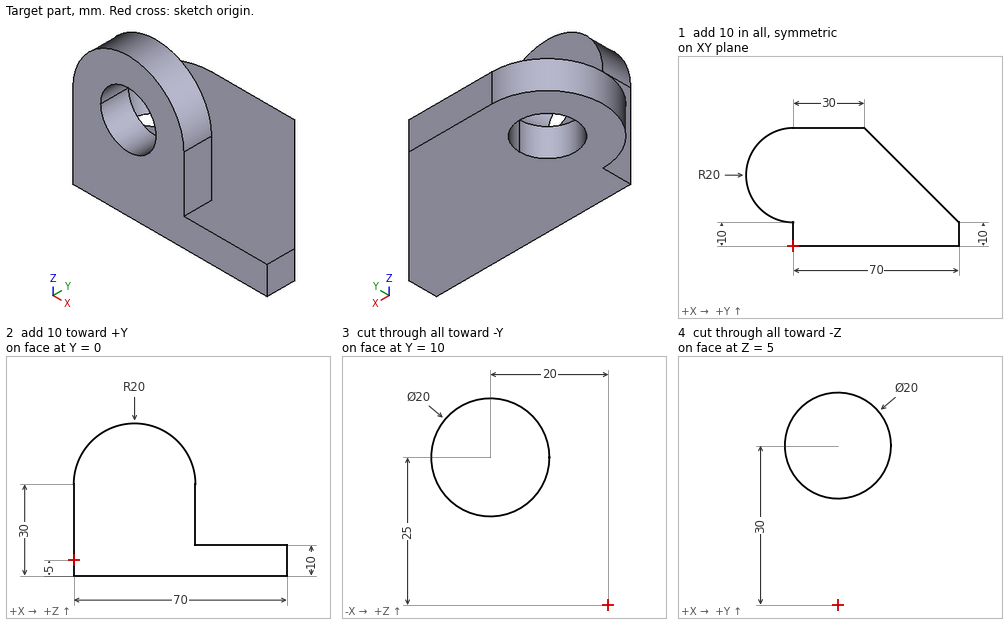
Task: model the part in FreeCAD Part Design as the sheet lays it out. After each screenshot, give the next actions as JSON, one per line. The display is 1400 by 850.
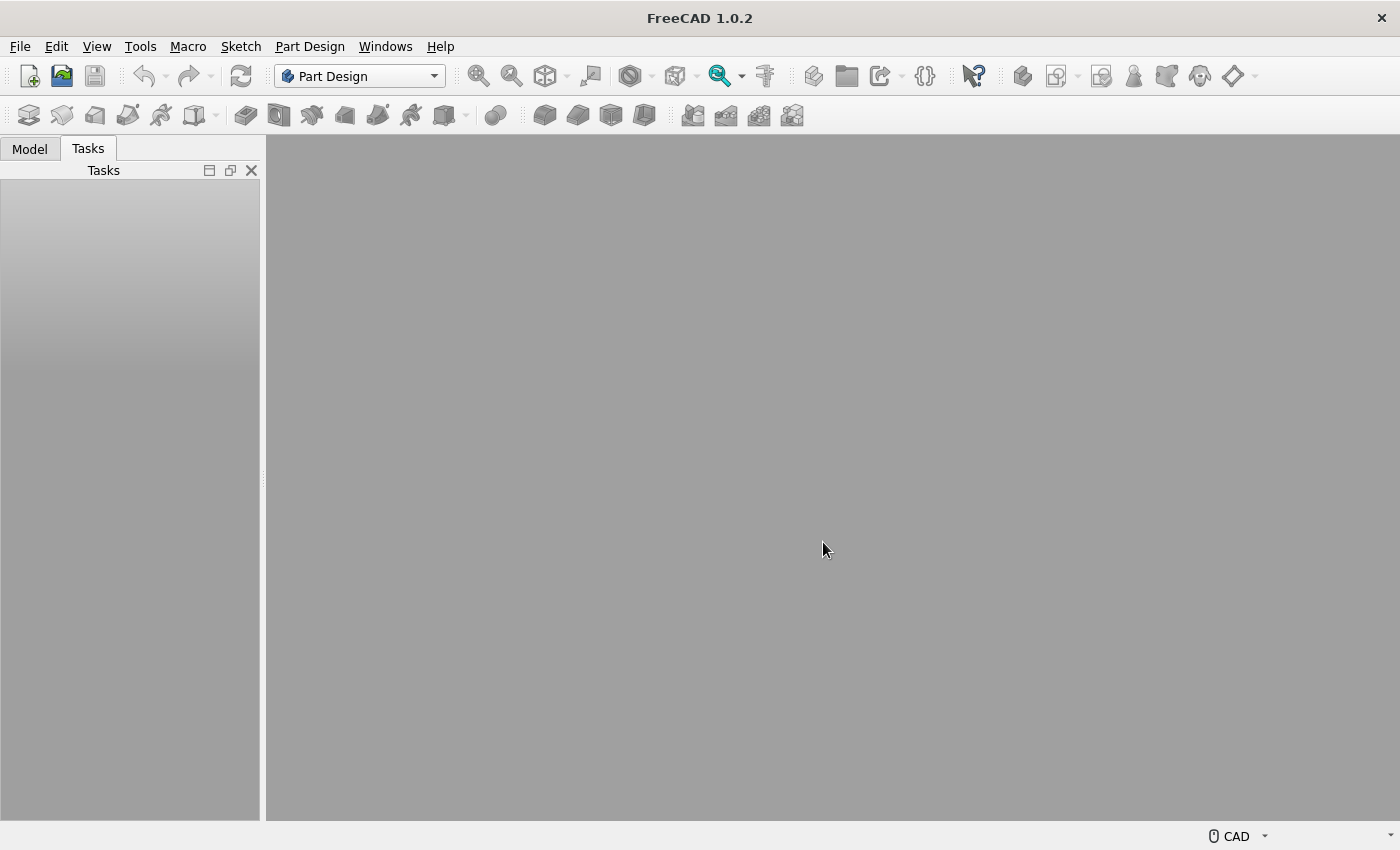
{"action": "left_click", "coordinate": [29, 76]}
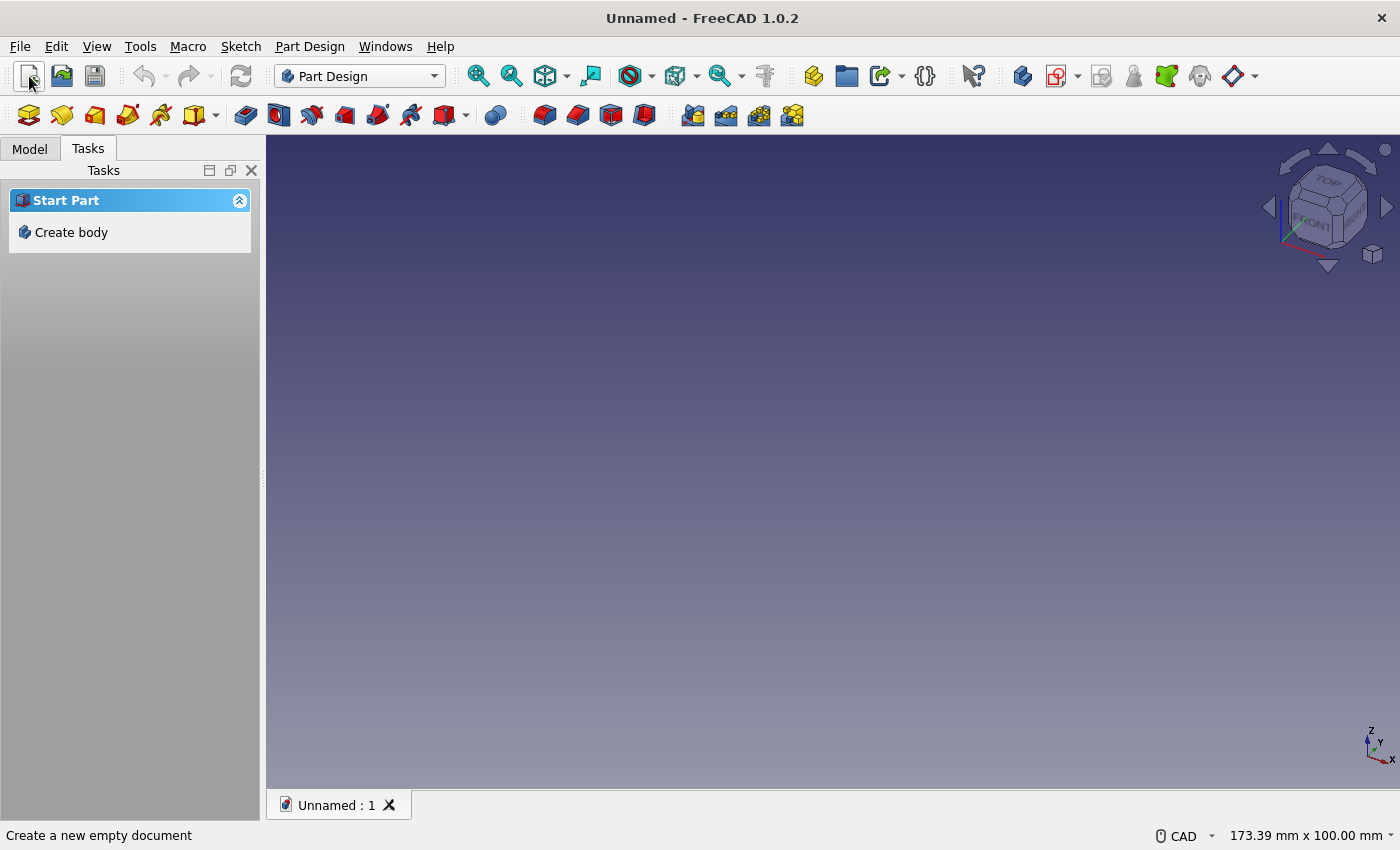
{"action": "left_click", "coordinate": [1056, 76]}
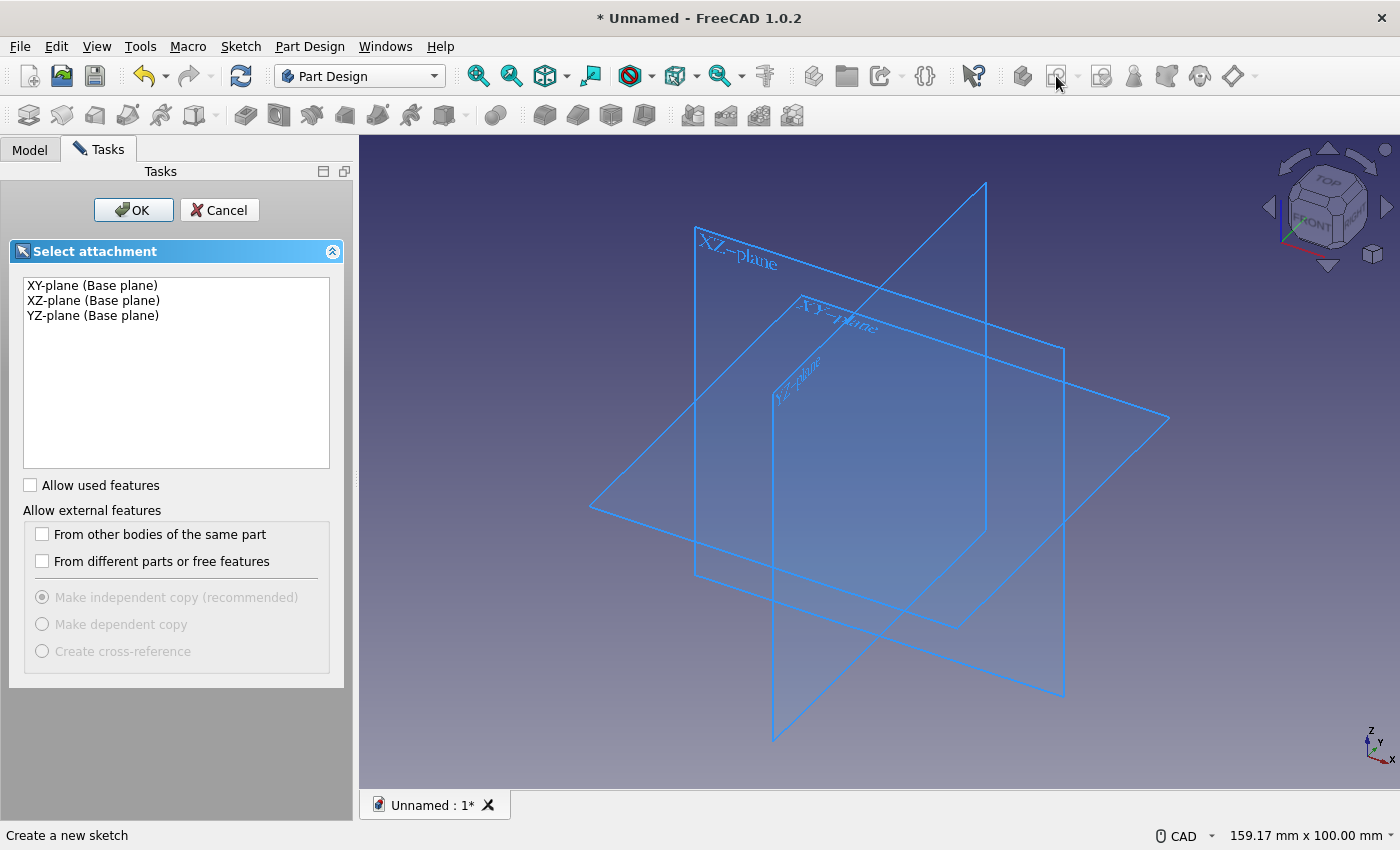
{"action": "left_click", "coordinate": [84, 286]}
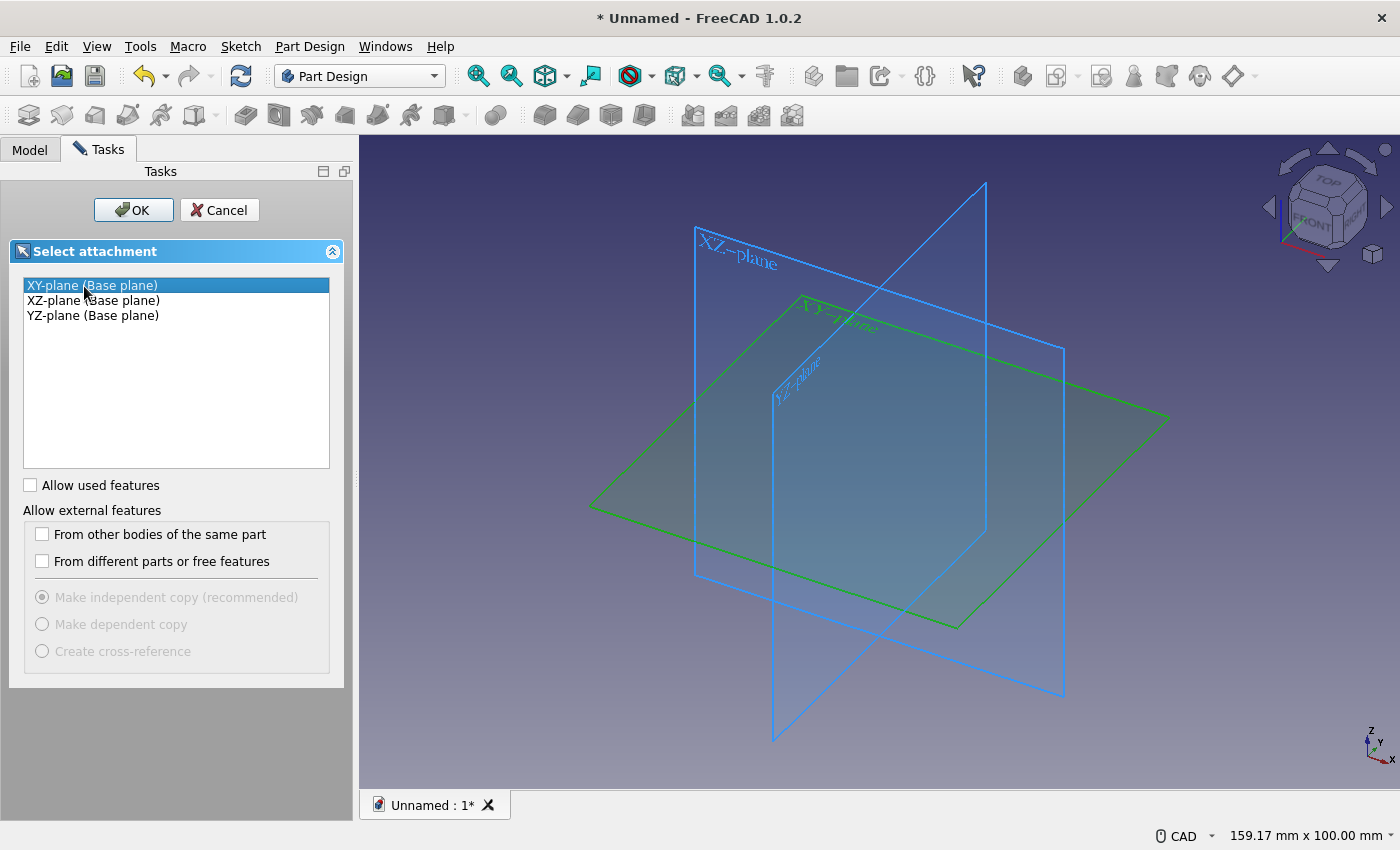
{"action": "left_click", "coordinate": [134, 210]}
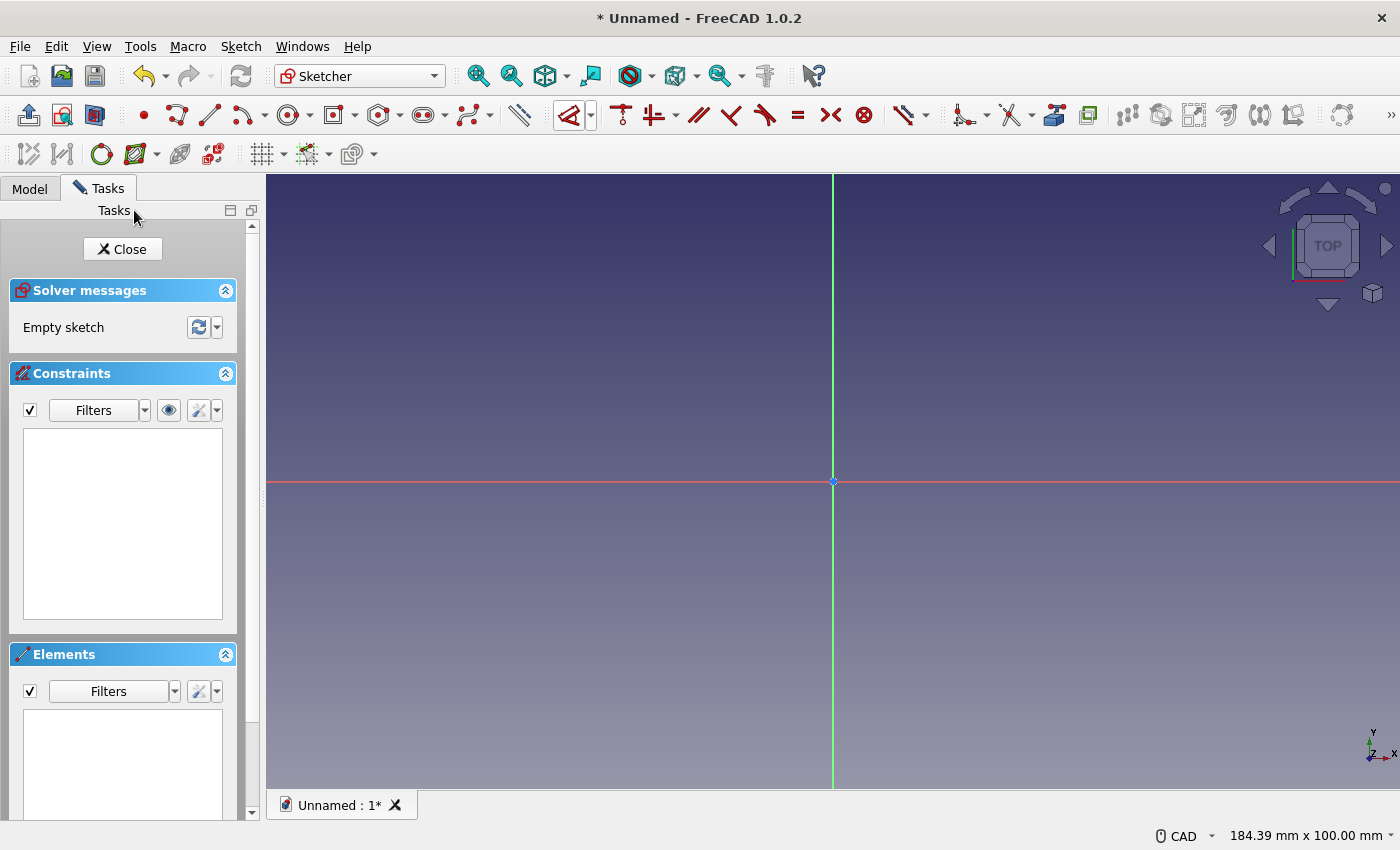
{"action": "scroll", "coordinate": [294, 761], "scroll_direction": "down", "scroll_amount": 1}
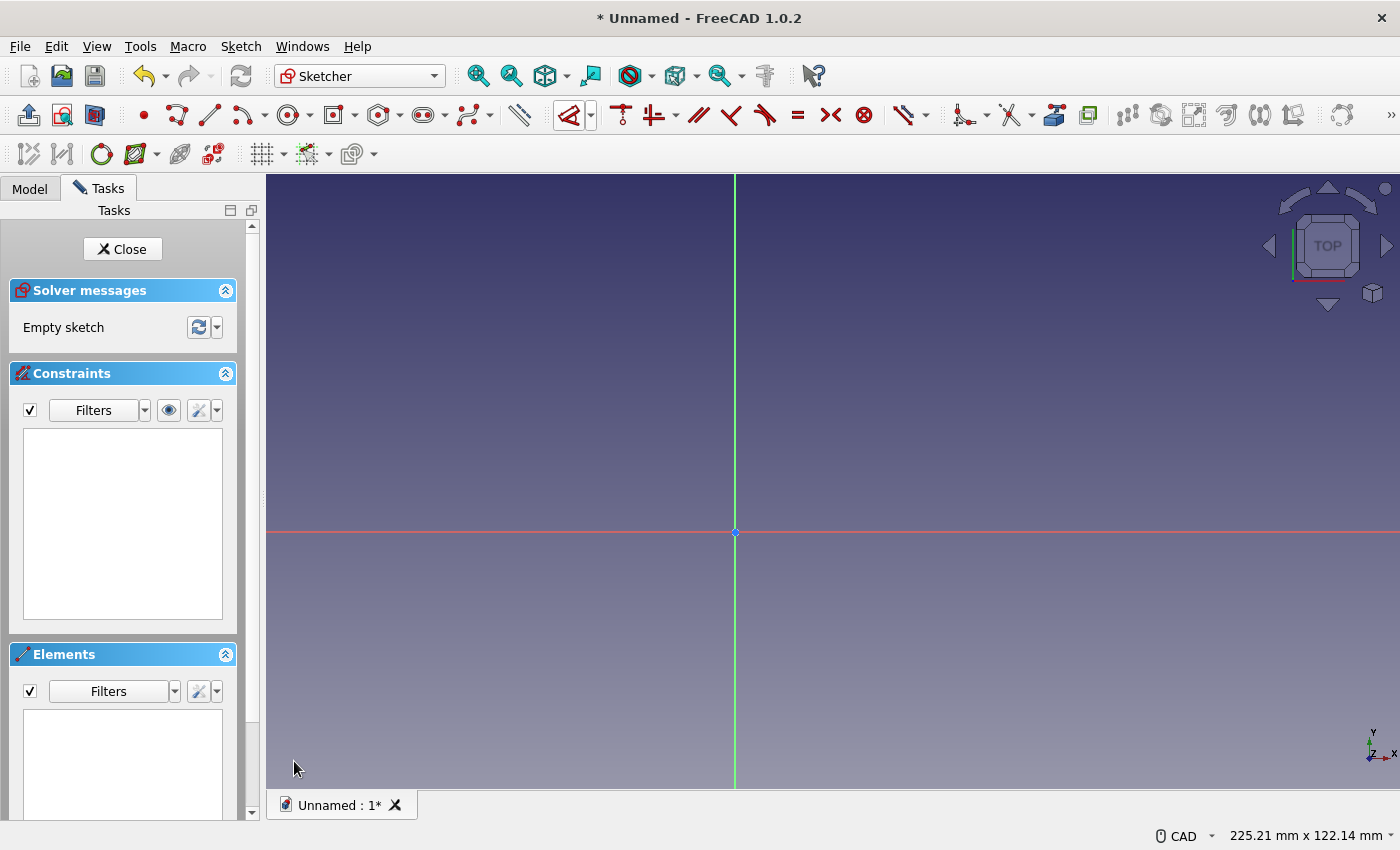
{"action": "scroll", "coordinate": [1058, 254], "scroll_direction": "up", "scroll_amount": 2}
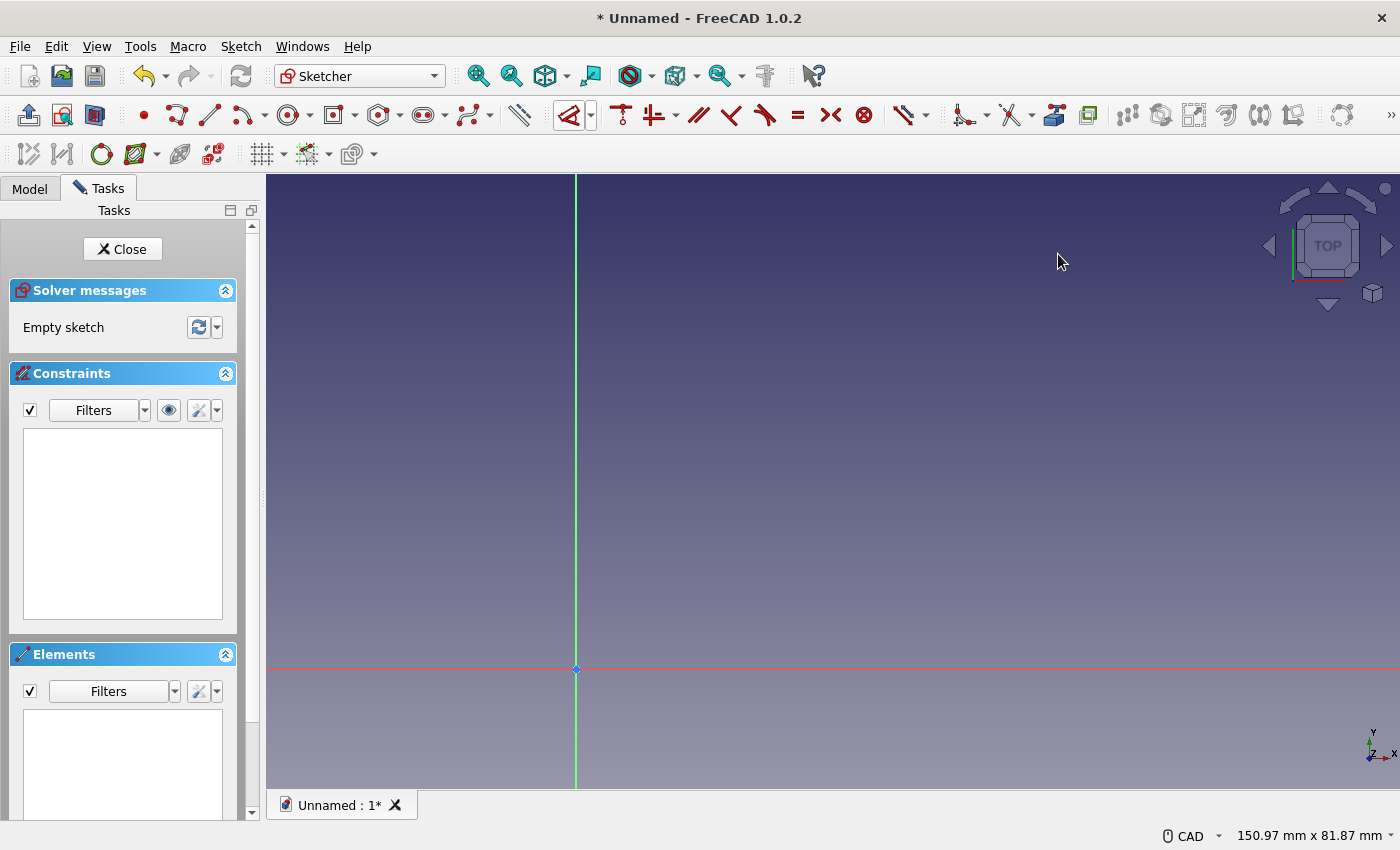
{"action": "left_click", "coordinate": [177, 116]}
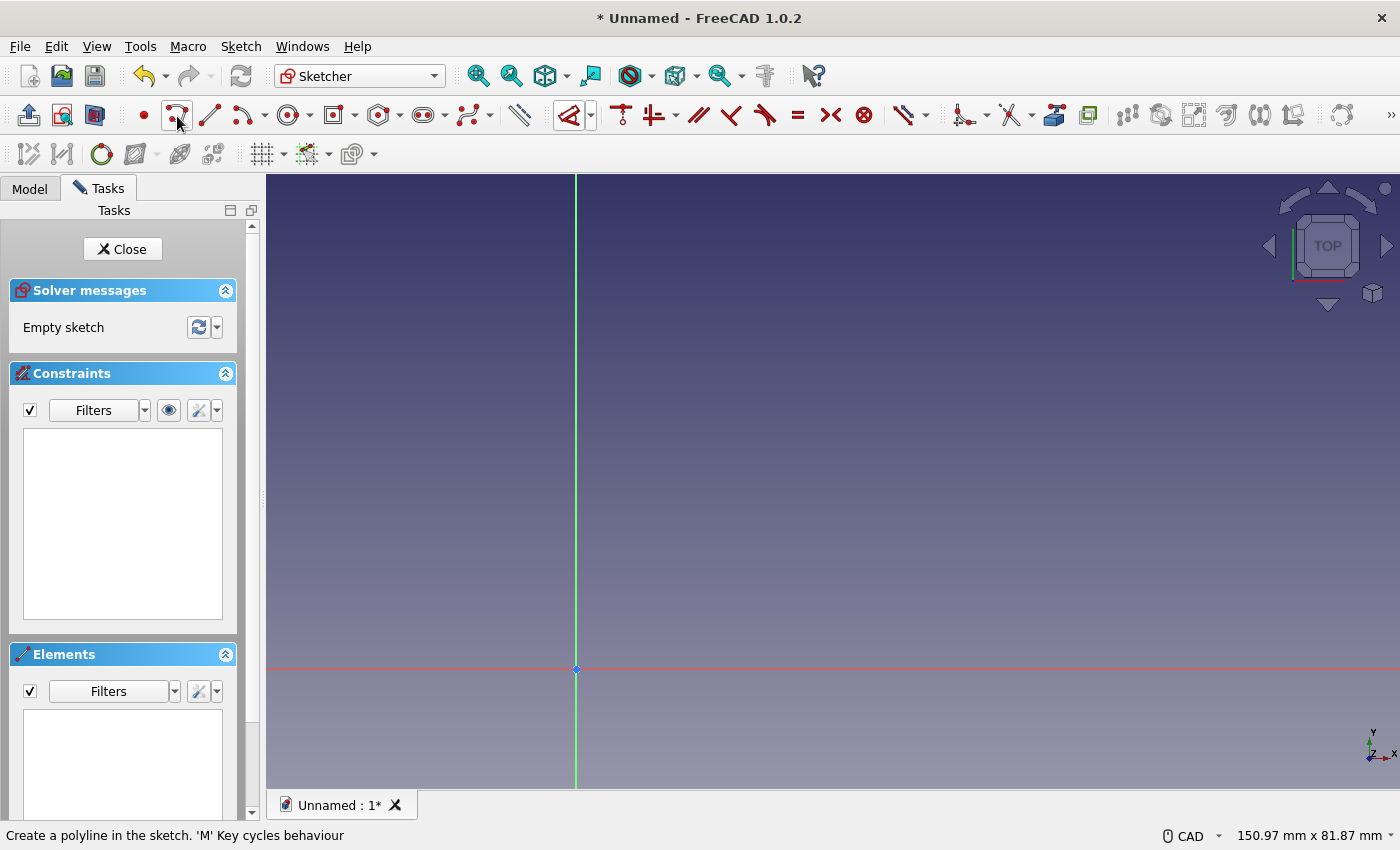
{"action": "left_click", "coordinate": [576, 594]}
{"action": "left_click", "coordinate": [576, 669]}
{"action": "left_click", "coordinate": [1102, 660]}
{"action": "left_click", "coordinate": [1102, 594]}
{"action": "left_click", "coordinate": [802, 294]}
{"action": "left_click", "coordinate": [576, 294]}
{"action": "right_click", "coordinate": [576, 294]}